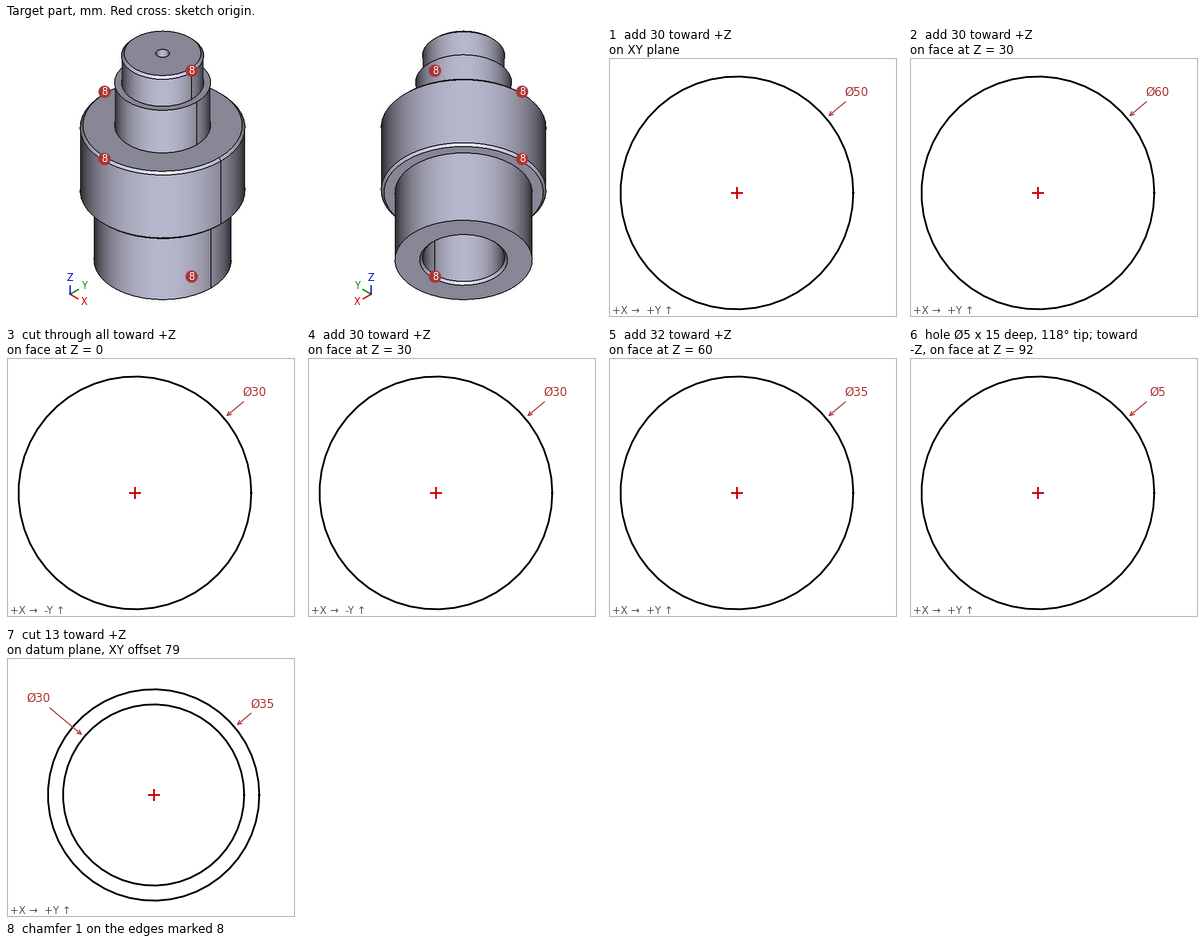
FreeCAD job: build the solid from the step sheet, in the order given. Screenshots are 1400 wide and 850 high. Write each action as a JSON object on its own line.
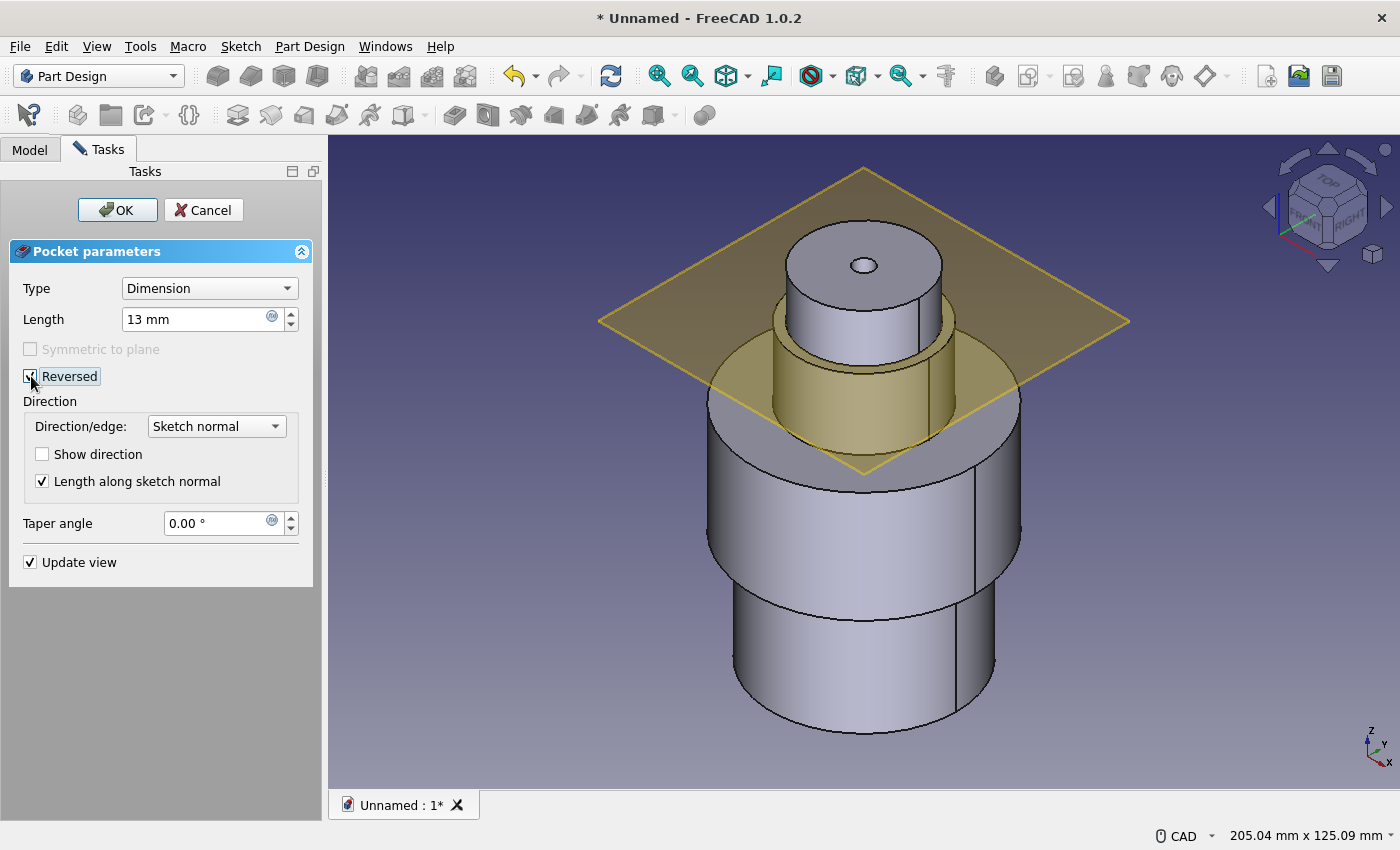
{"action": "left_click", "coordinate": [118, 210]}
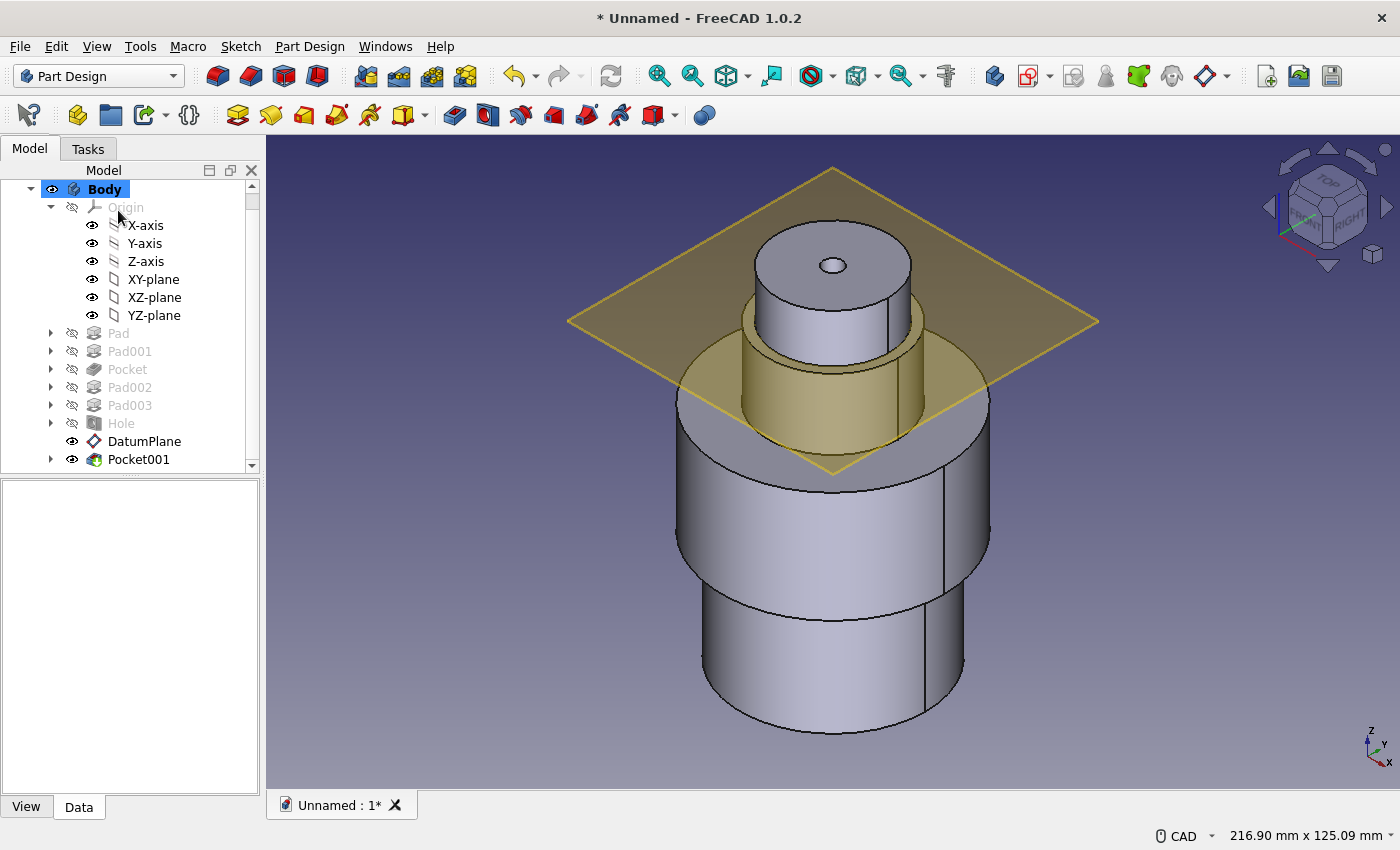
{"action": "left_click", "coordinate": [117, 441]}
{"action": "key", "text": "space"}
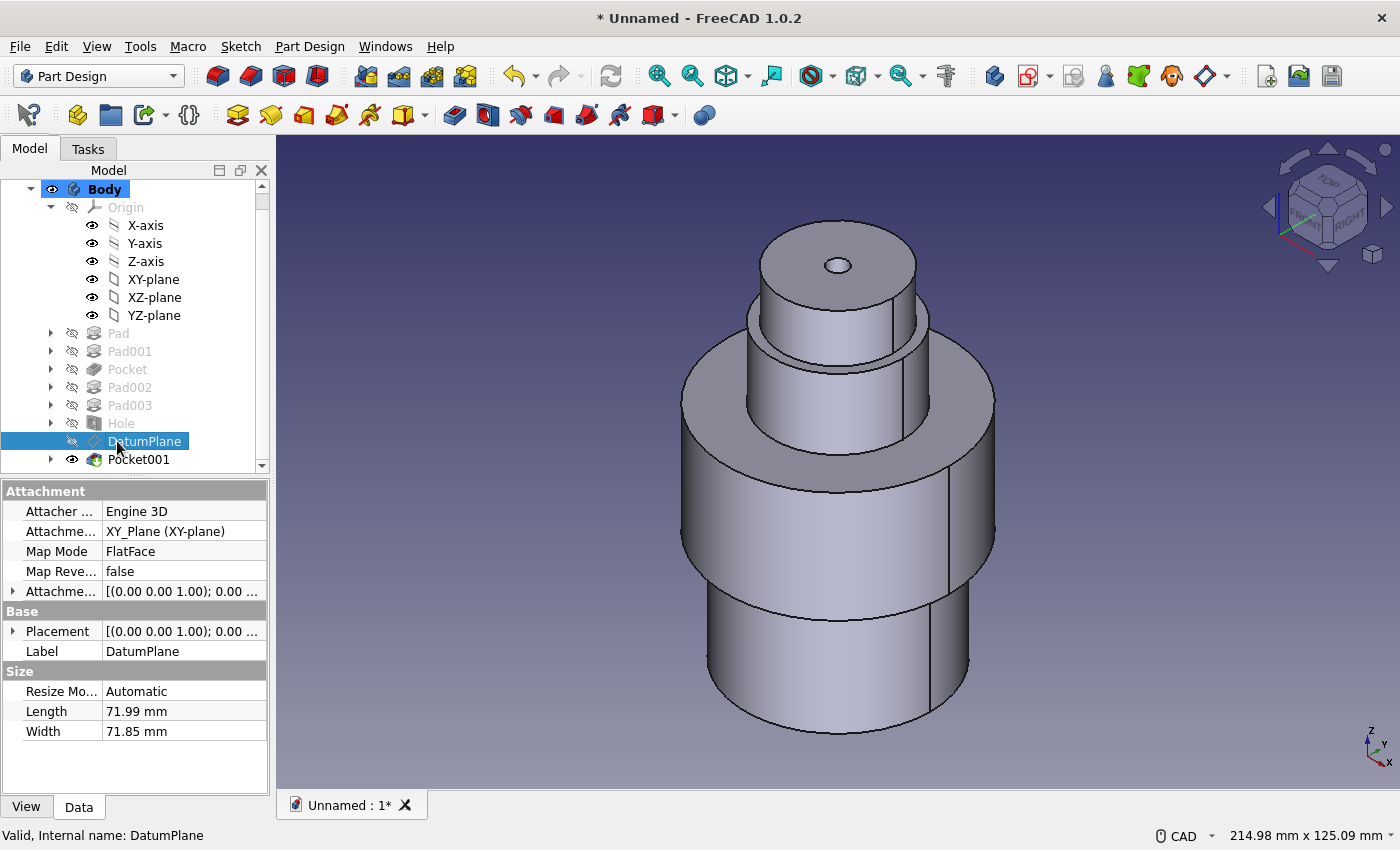
{"action": "left_click", "coordinate": [761, 258]}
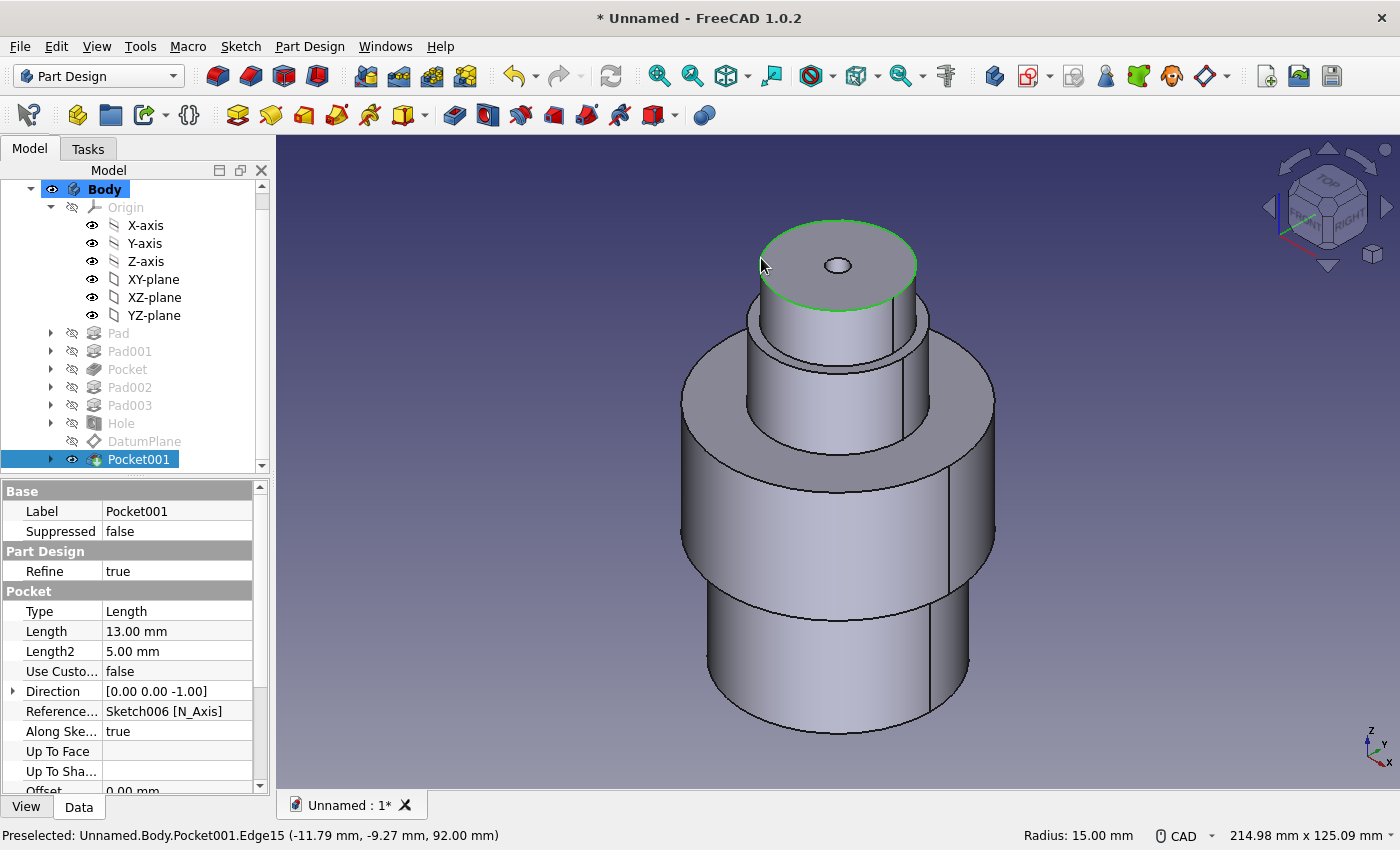
{"action": "left_click", "coordinate": [698, 442], "text": "ctrl"}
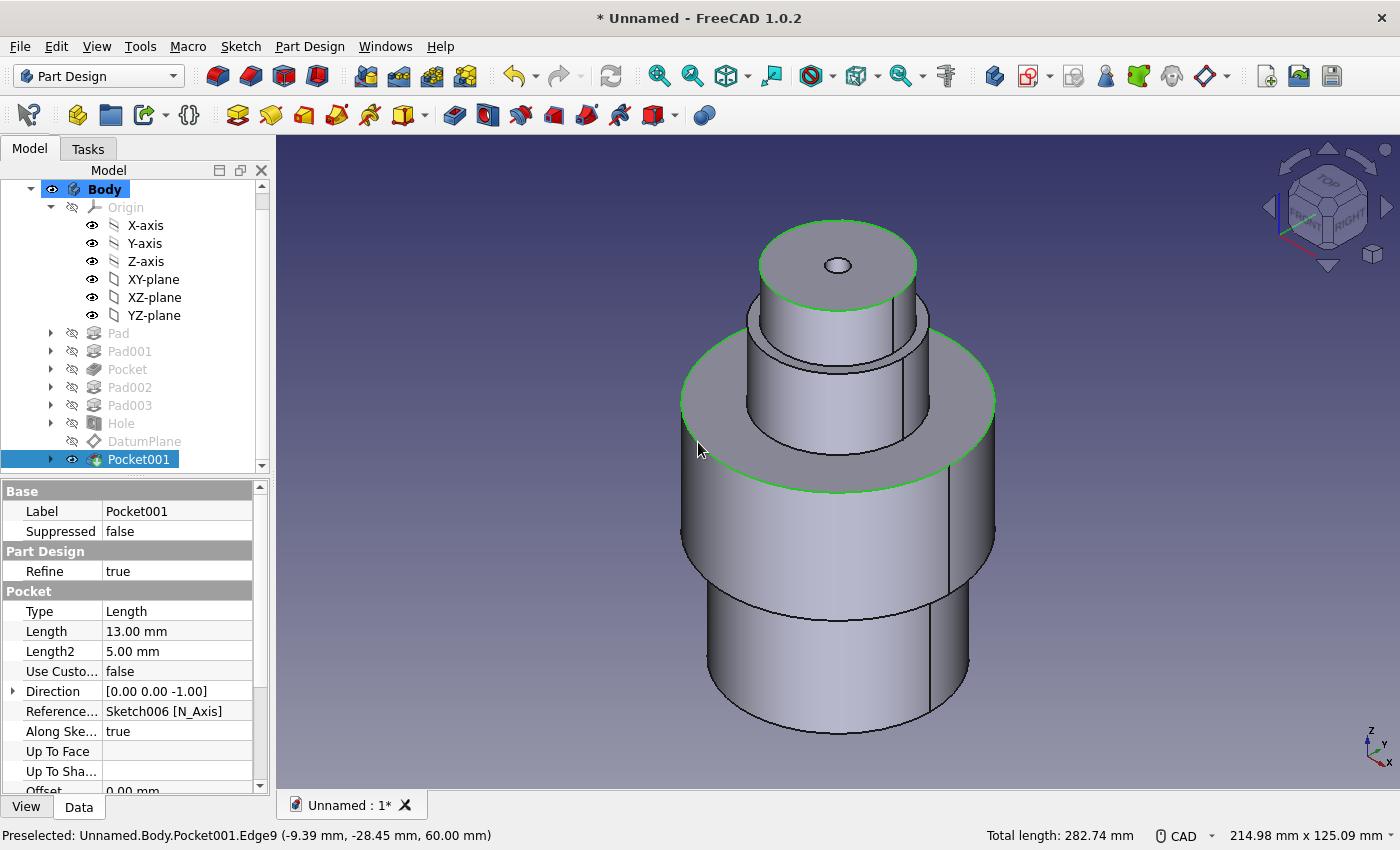
{"action": "key", "text": "2"}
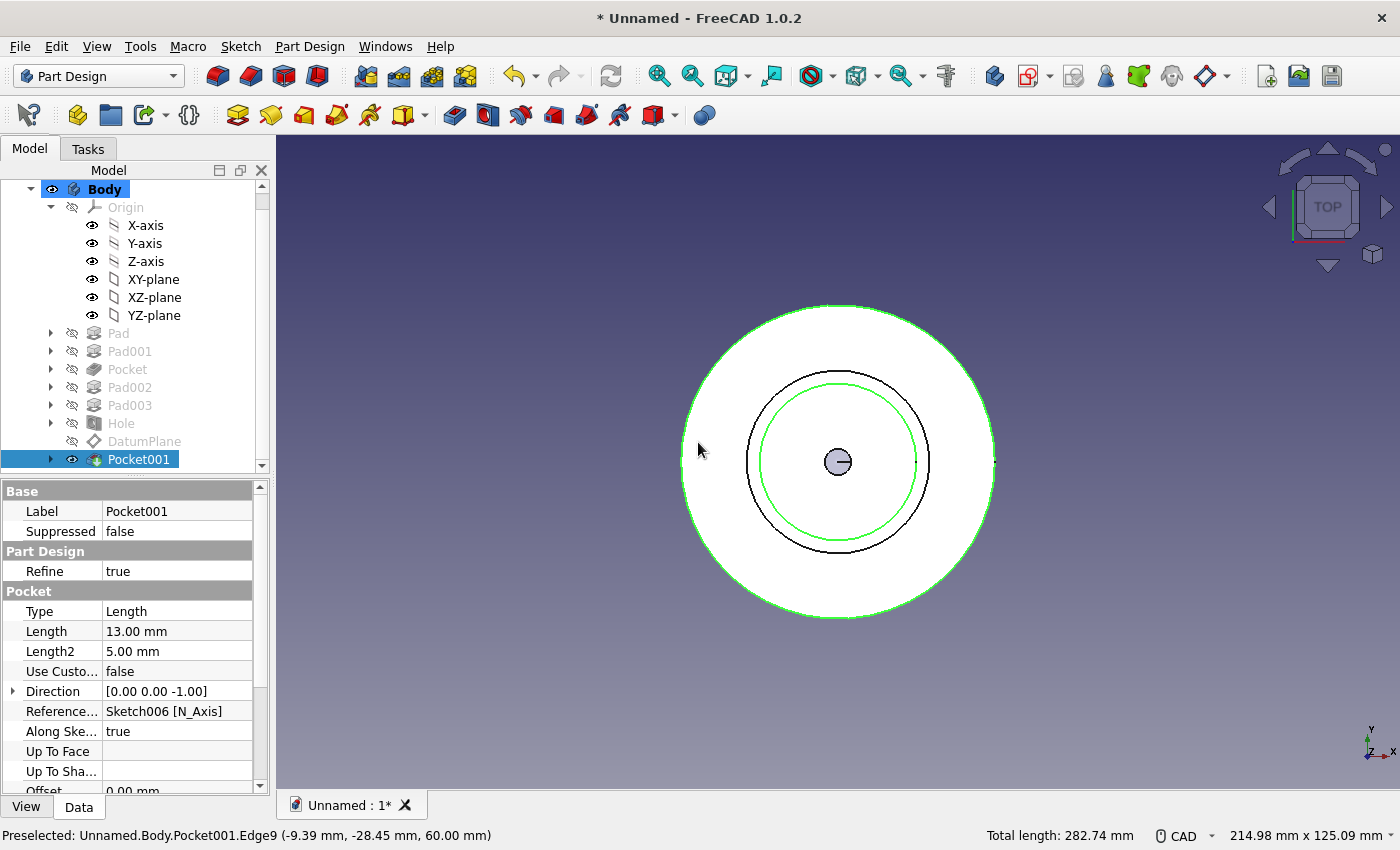
{"action": "key", "text": "0"}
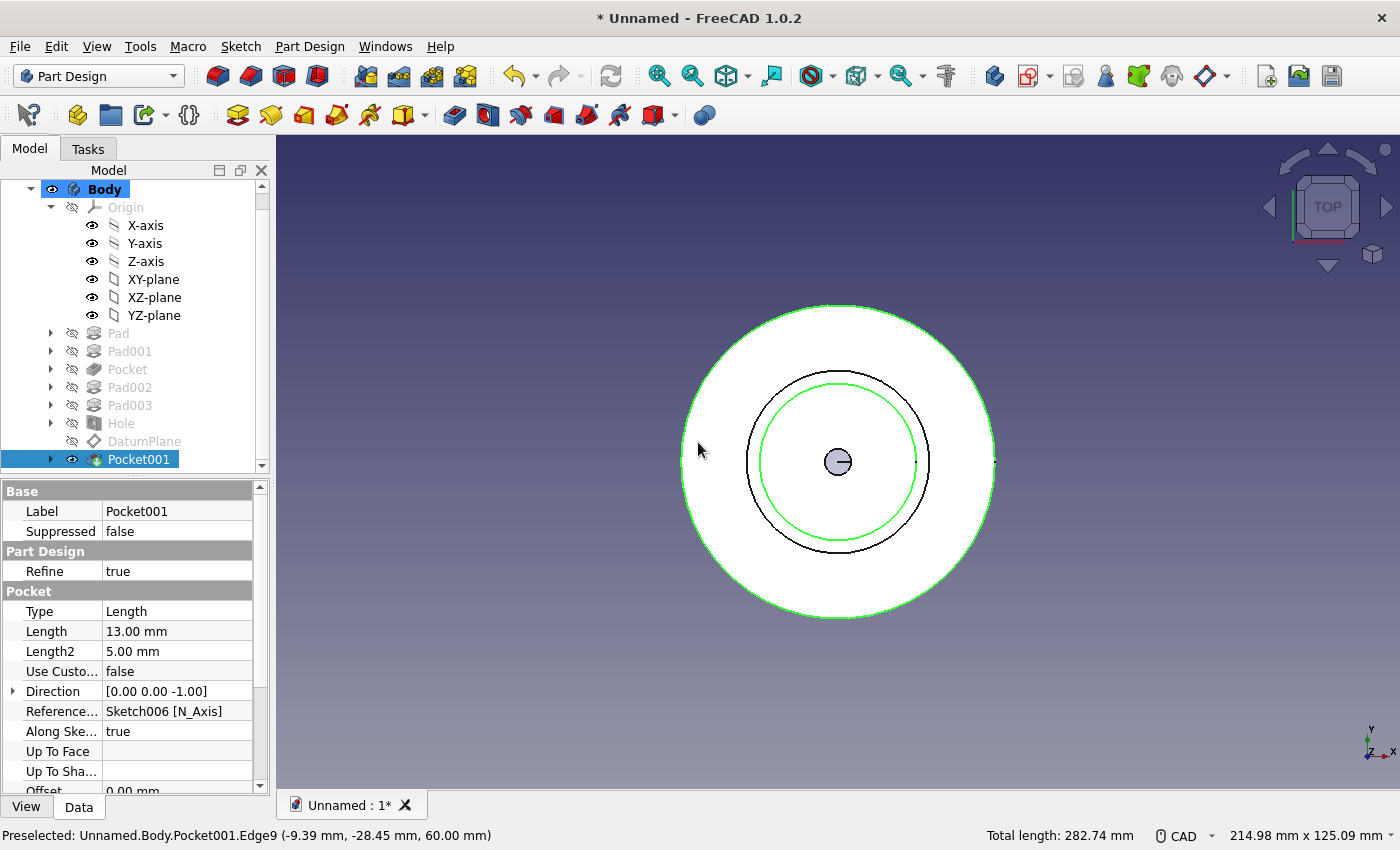
{"action": "key", "text": "1"}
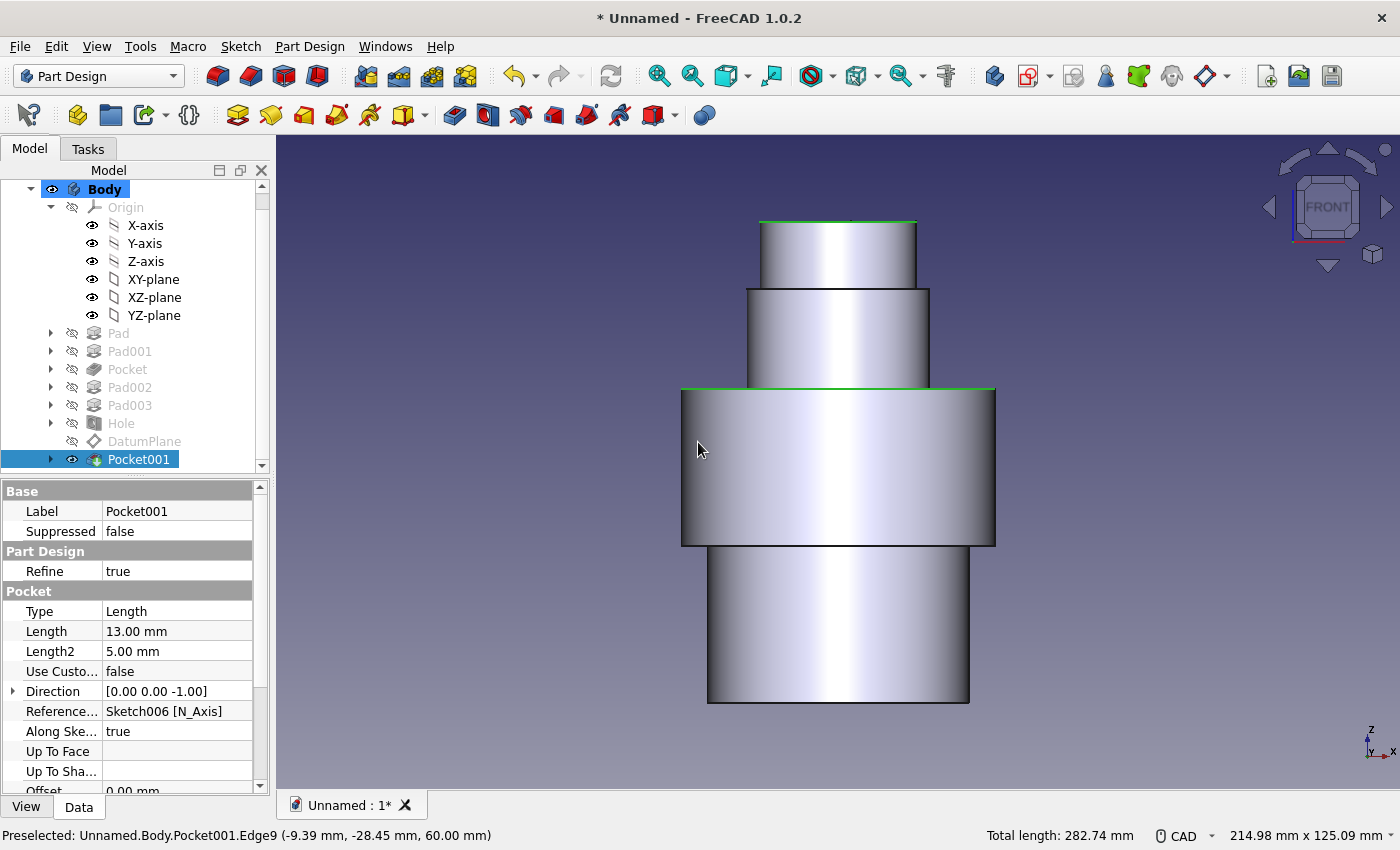
{"action": "left_click", "coordinate": [711, 545], "text": "ctrl"}